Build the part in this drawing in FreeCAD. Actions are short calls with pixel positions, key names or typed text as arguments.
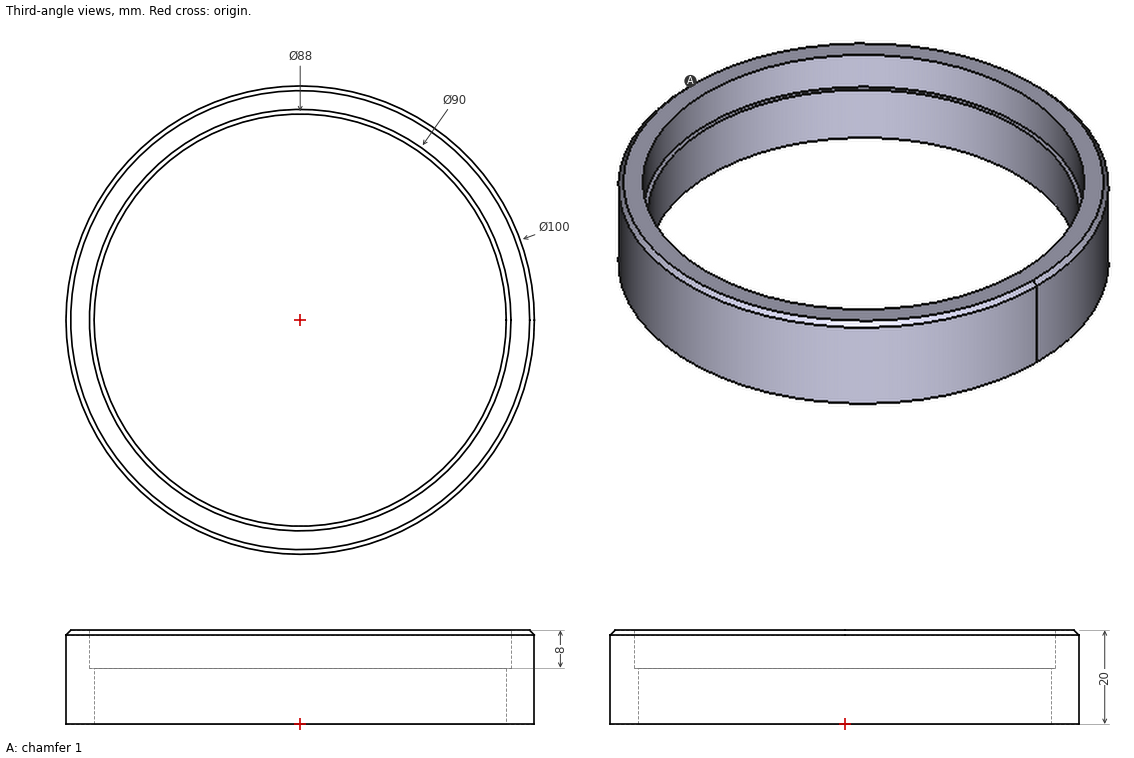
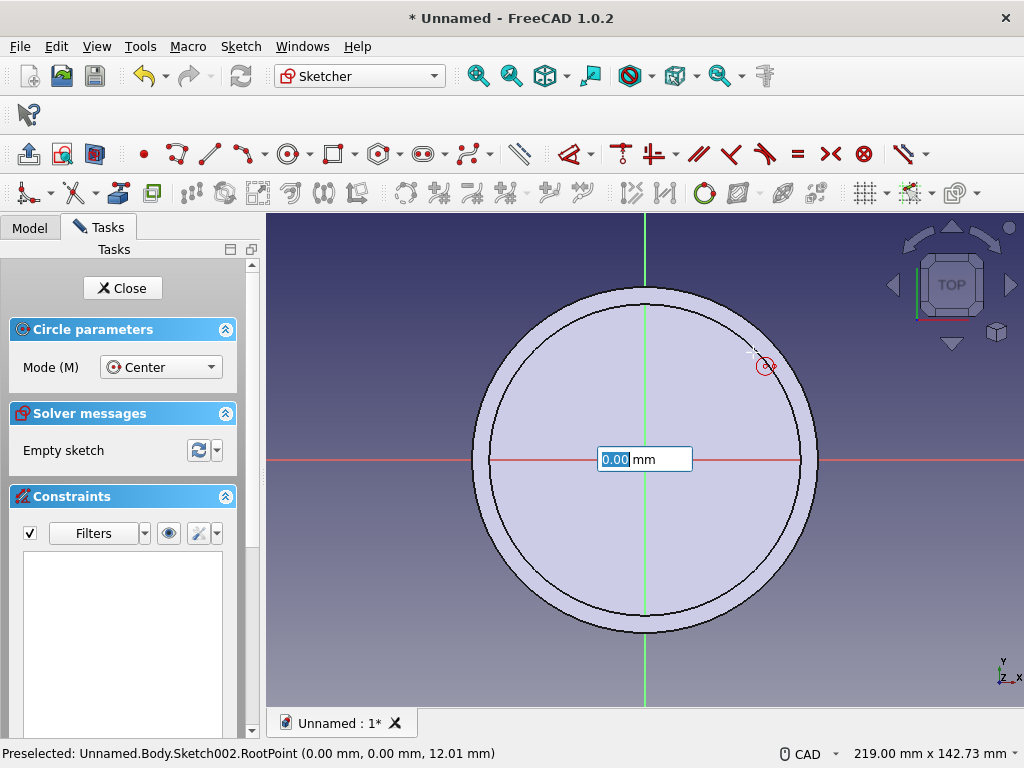
text(88)
key(Return)
key(Escape)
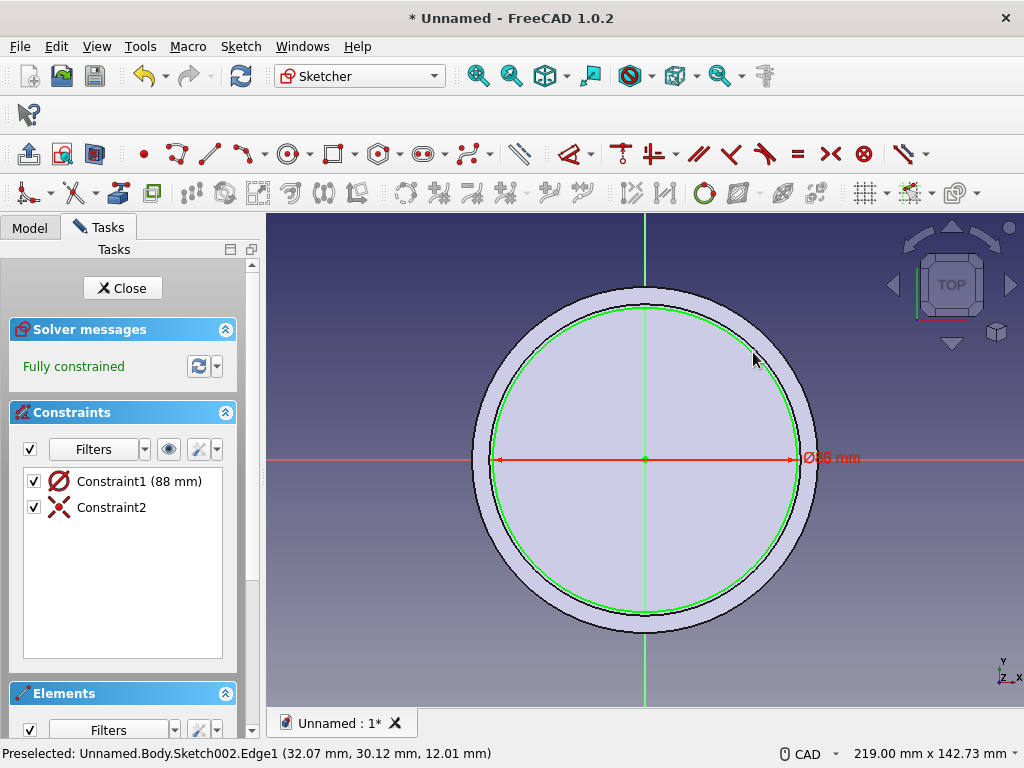
click(123, 288)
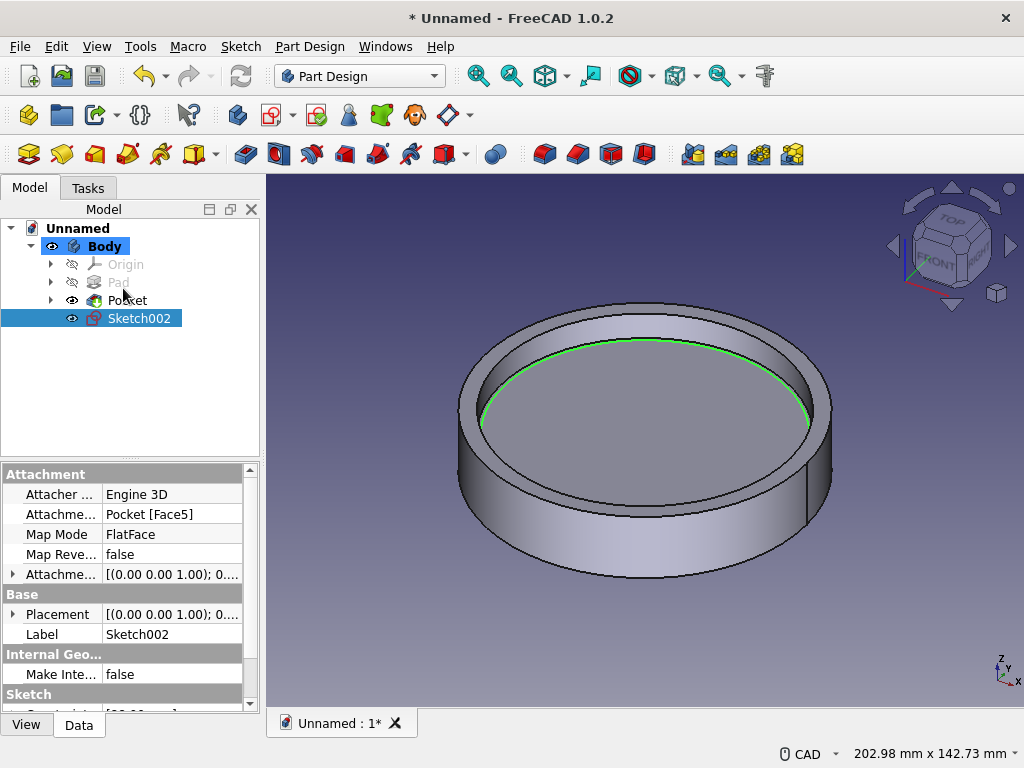
click(246, 154)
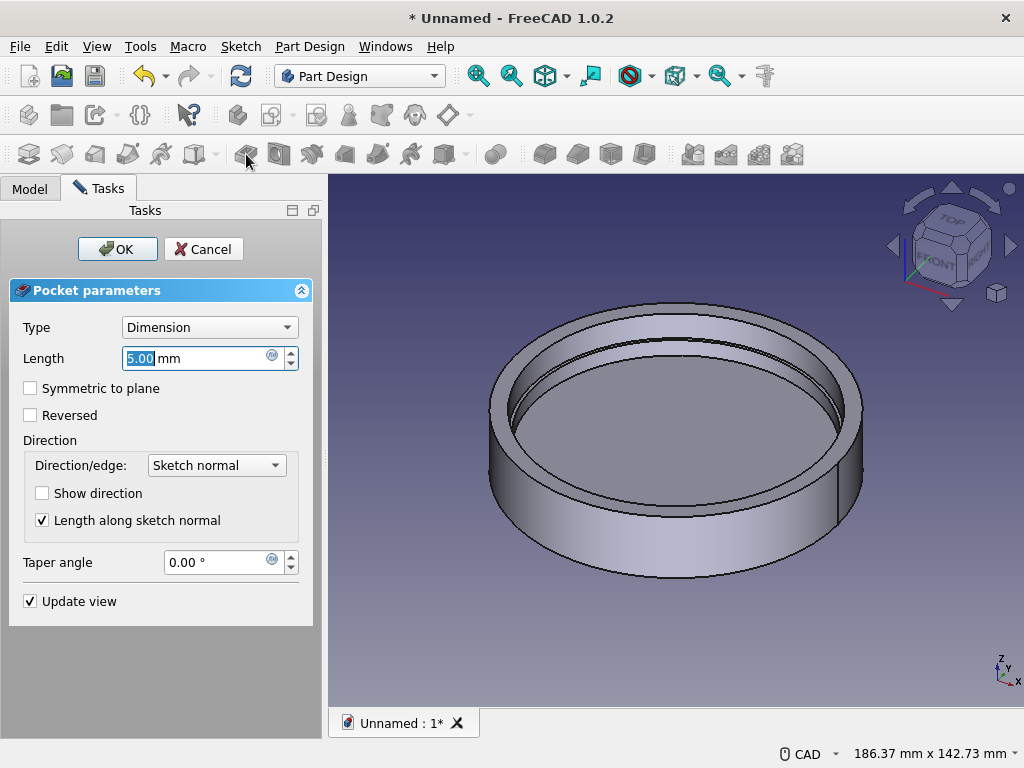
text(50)
key(Tab)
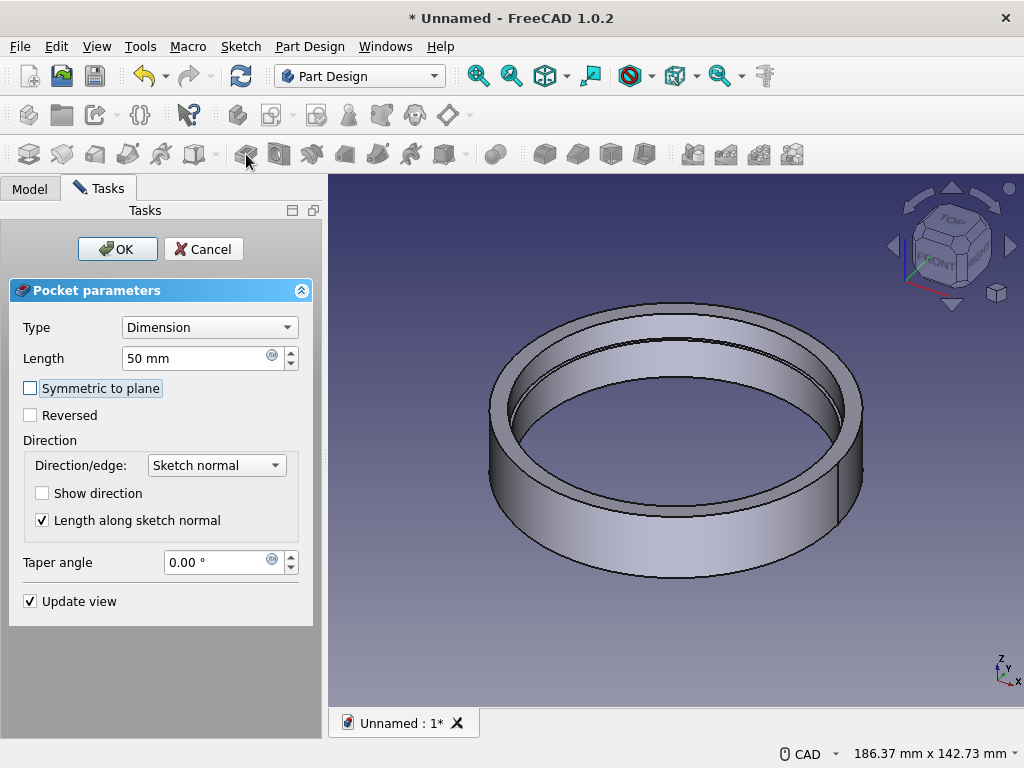
click(118, 249)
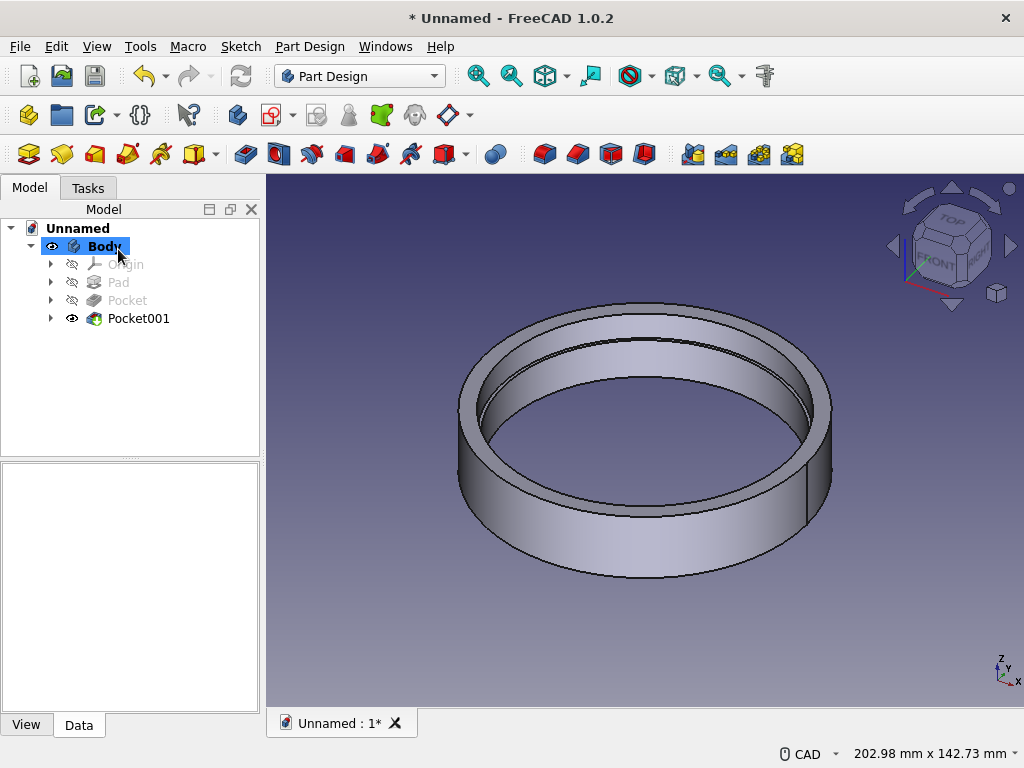
click(459, 420)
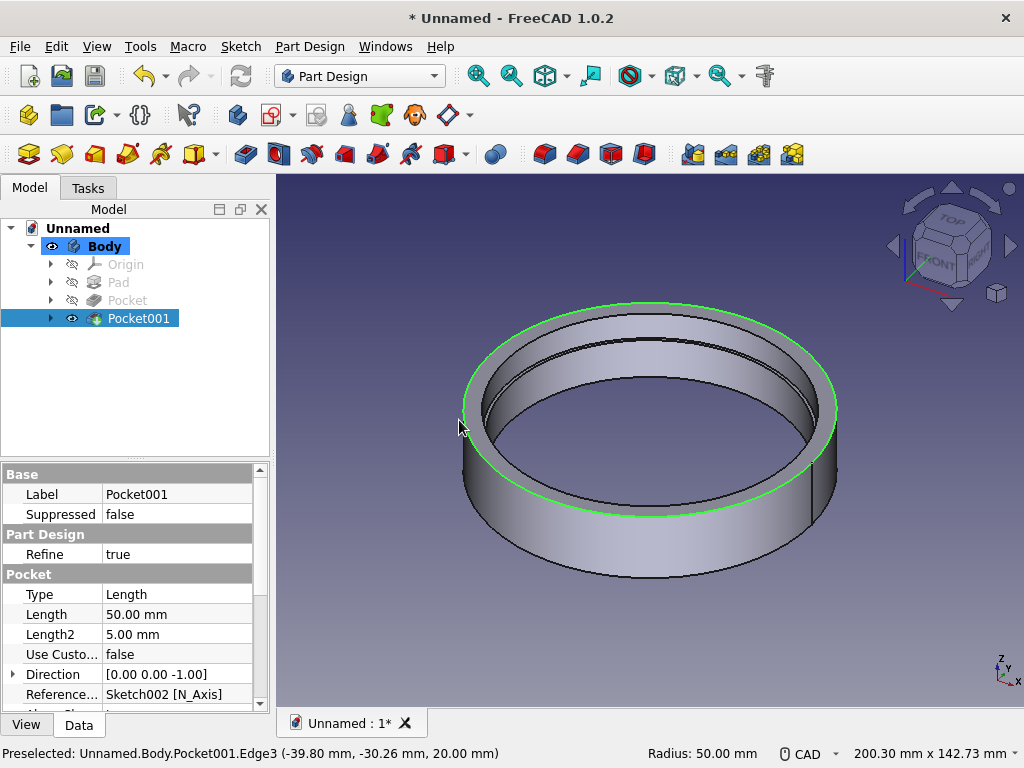
click(578, 154)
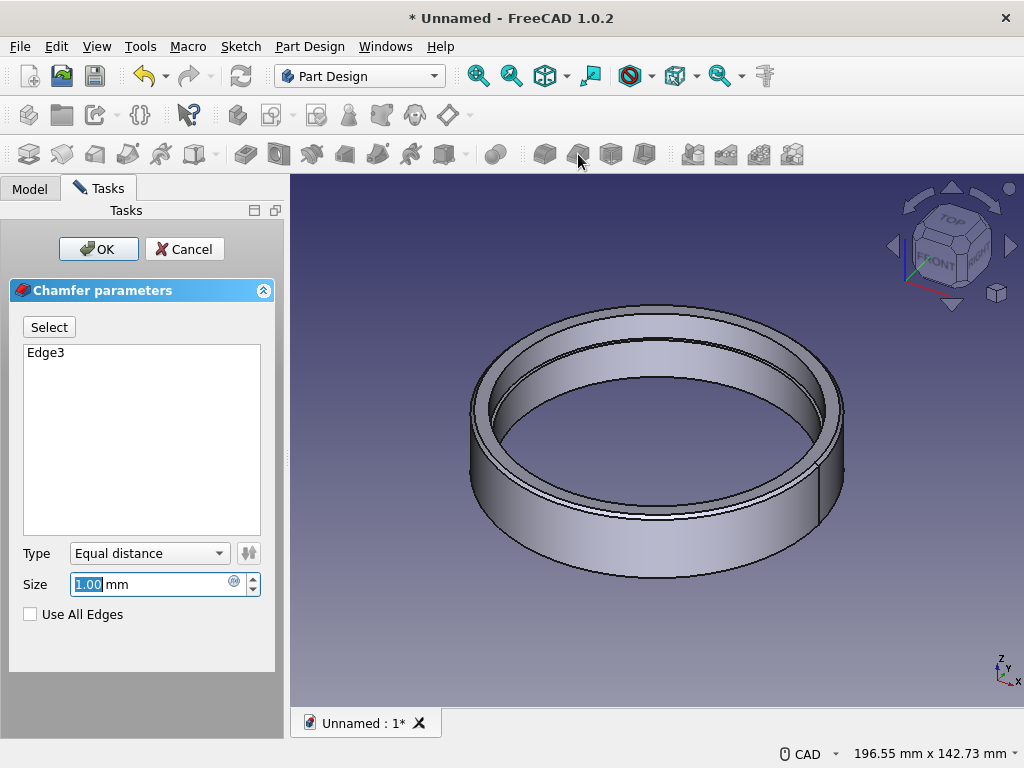
text(1)
key(Tab)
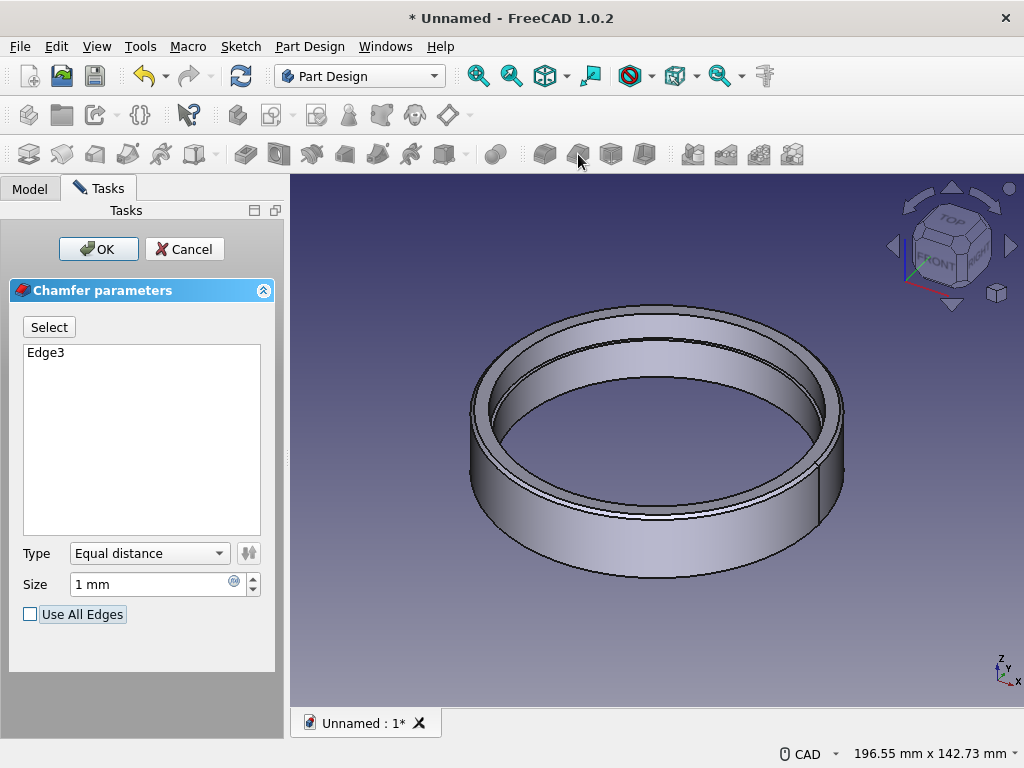
click(99, 249)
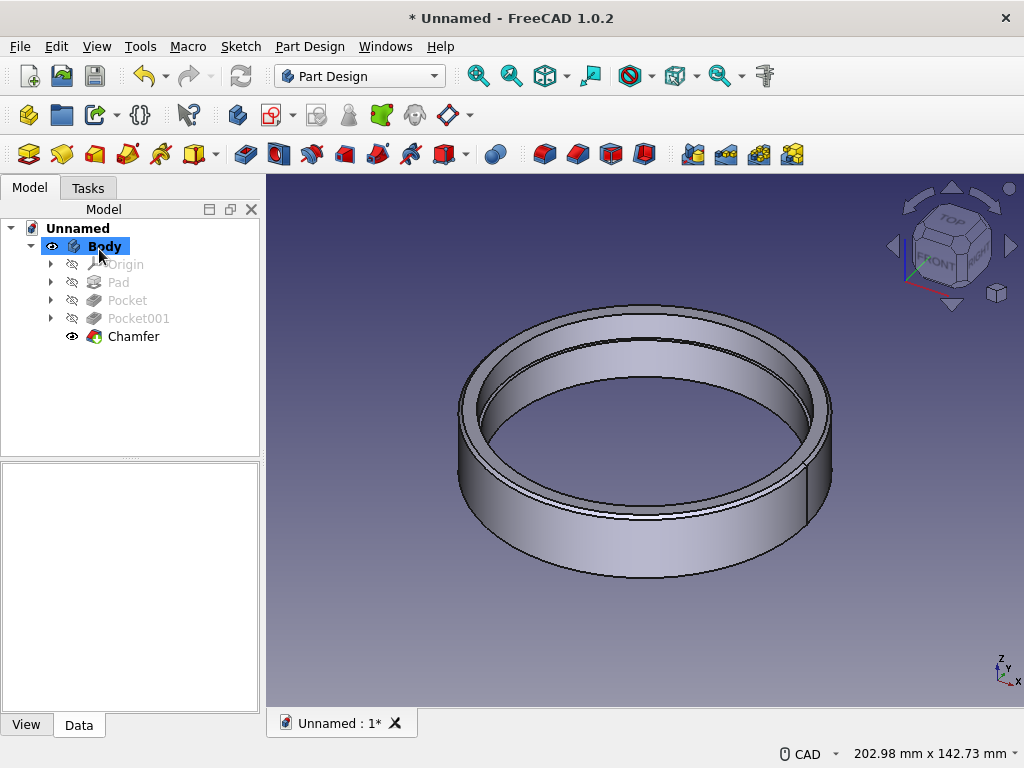
key(0)